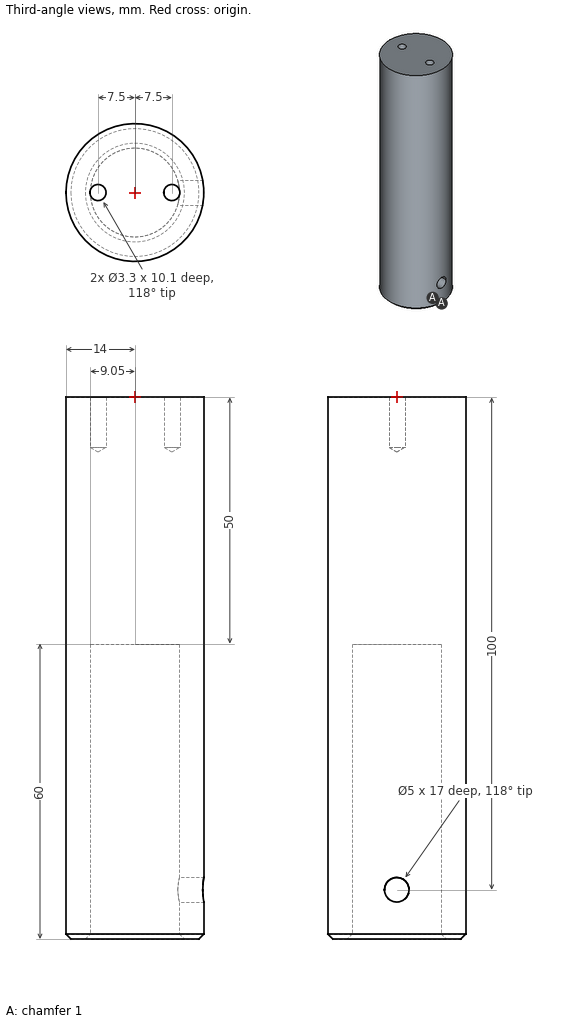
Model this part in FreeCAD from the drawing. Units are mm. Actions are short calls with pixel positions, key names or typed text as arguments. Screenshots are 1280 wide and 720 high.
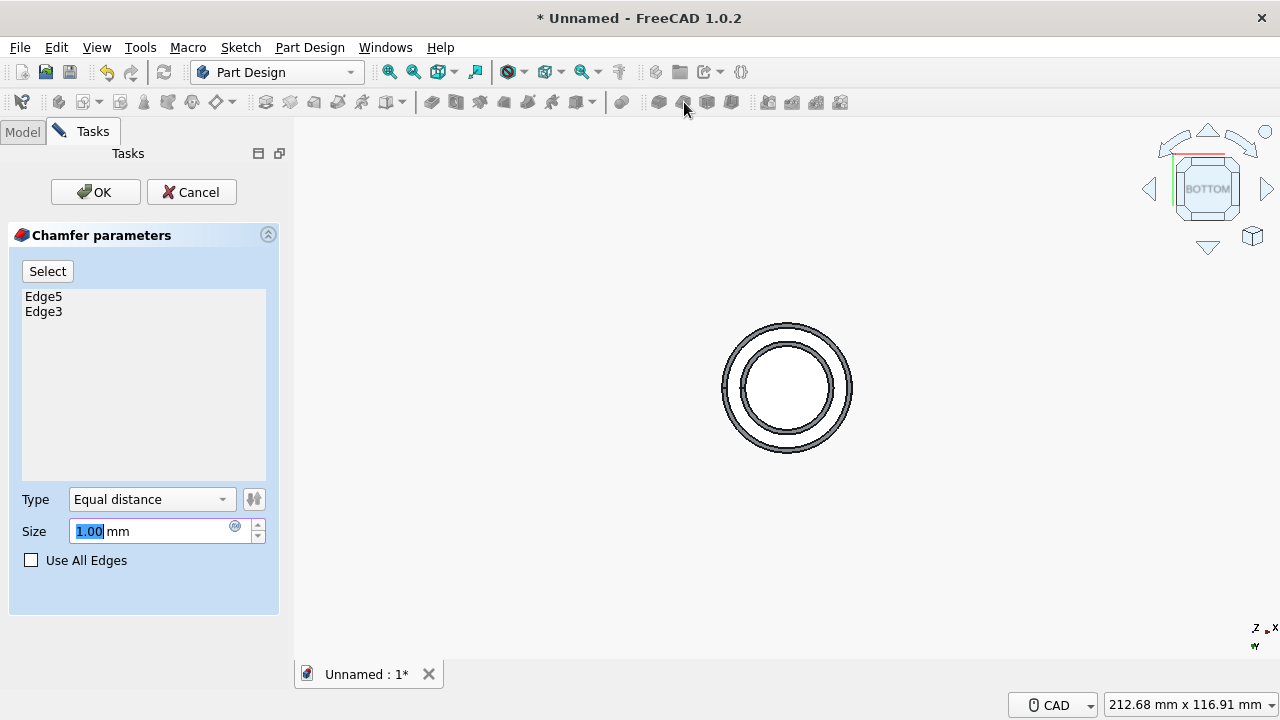
text(1)
key(Tab)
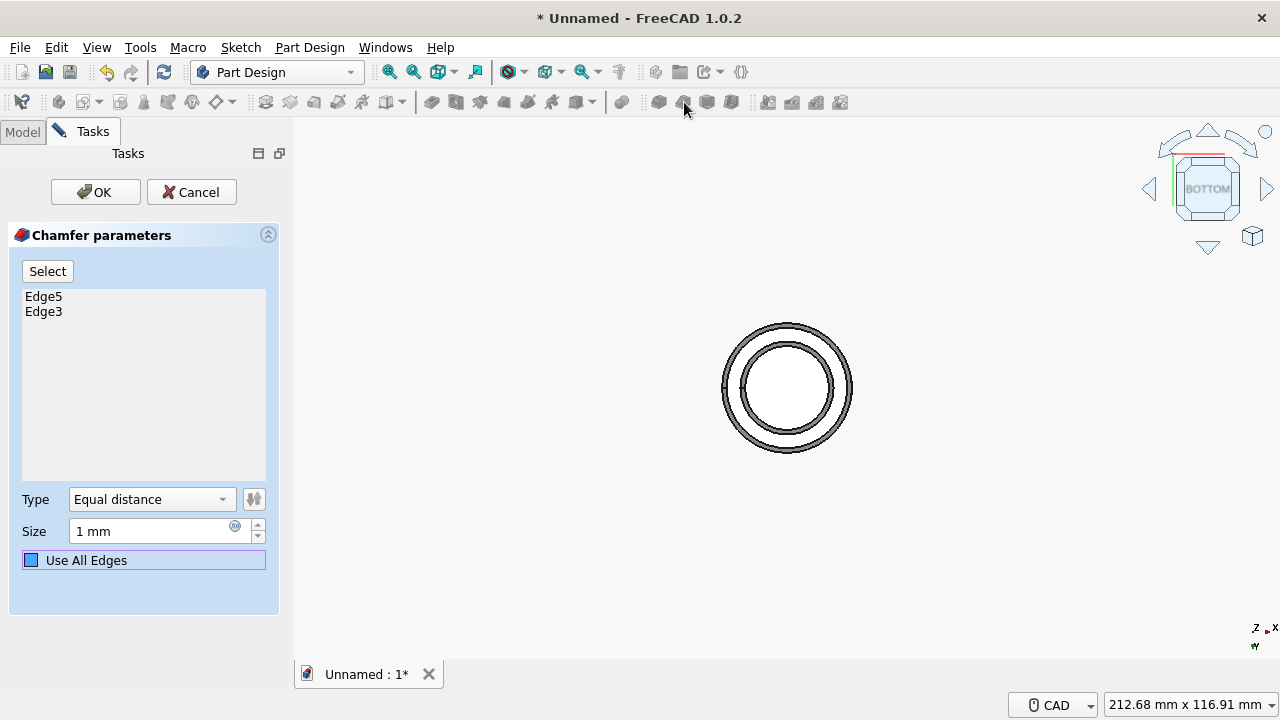
click(96, 192)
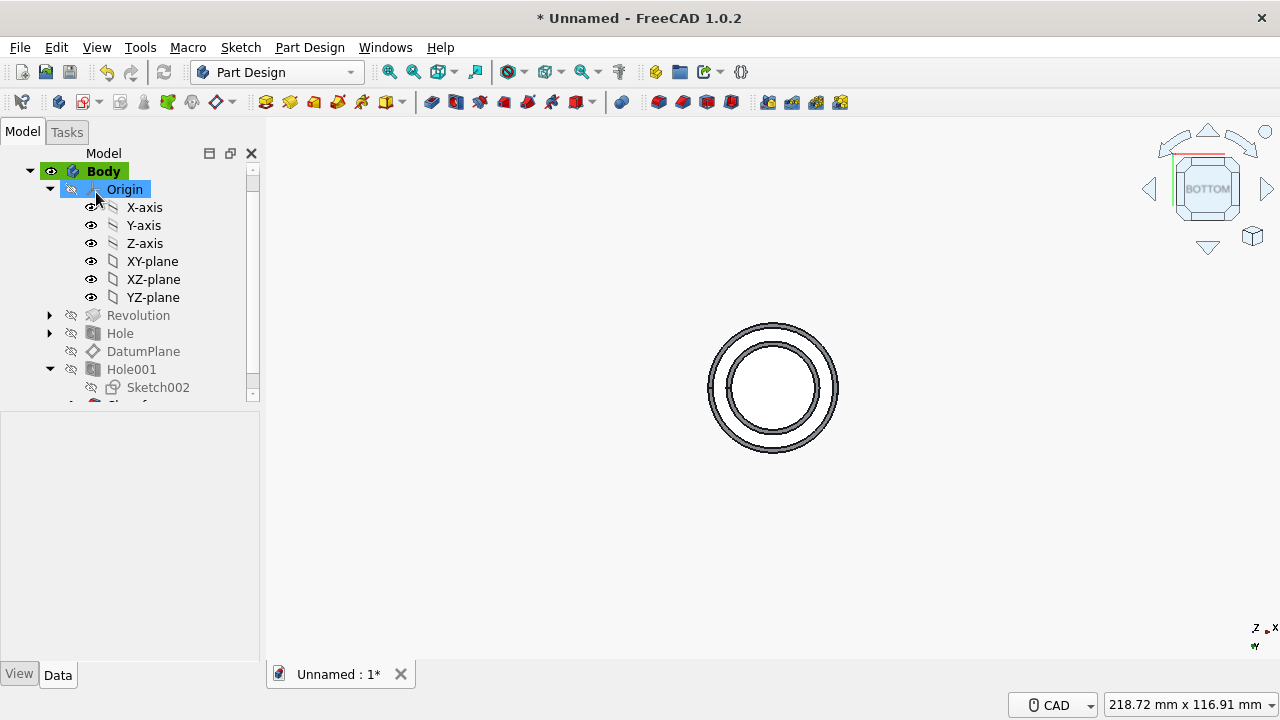
key(0)